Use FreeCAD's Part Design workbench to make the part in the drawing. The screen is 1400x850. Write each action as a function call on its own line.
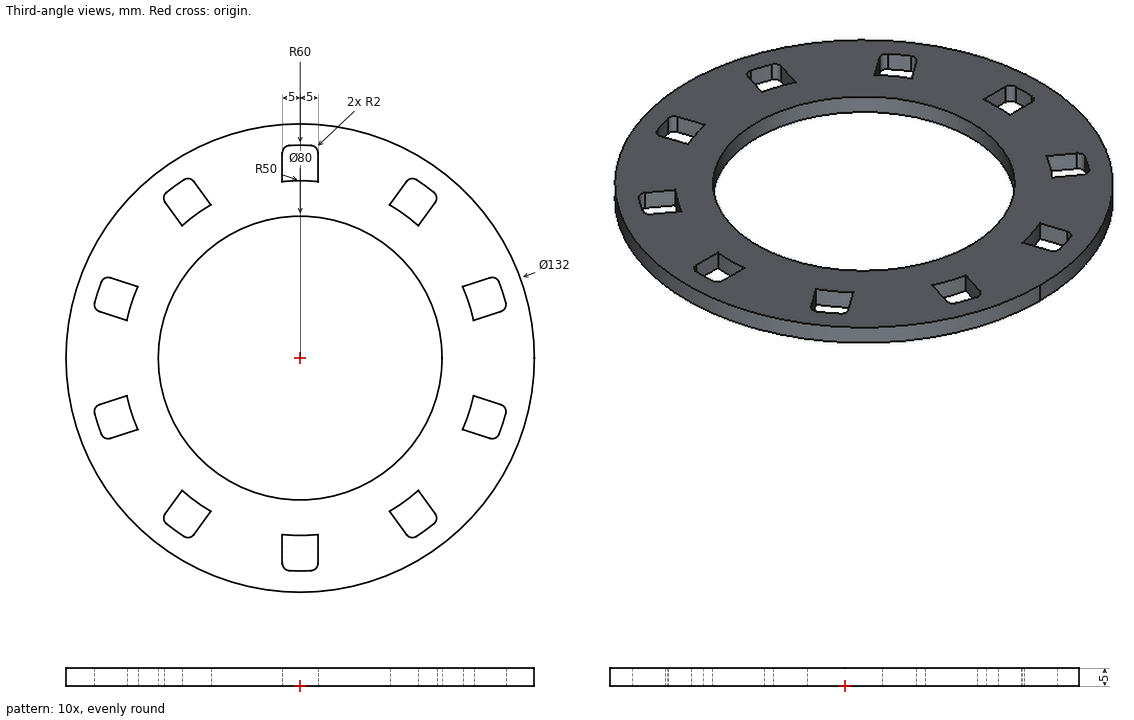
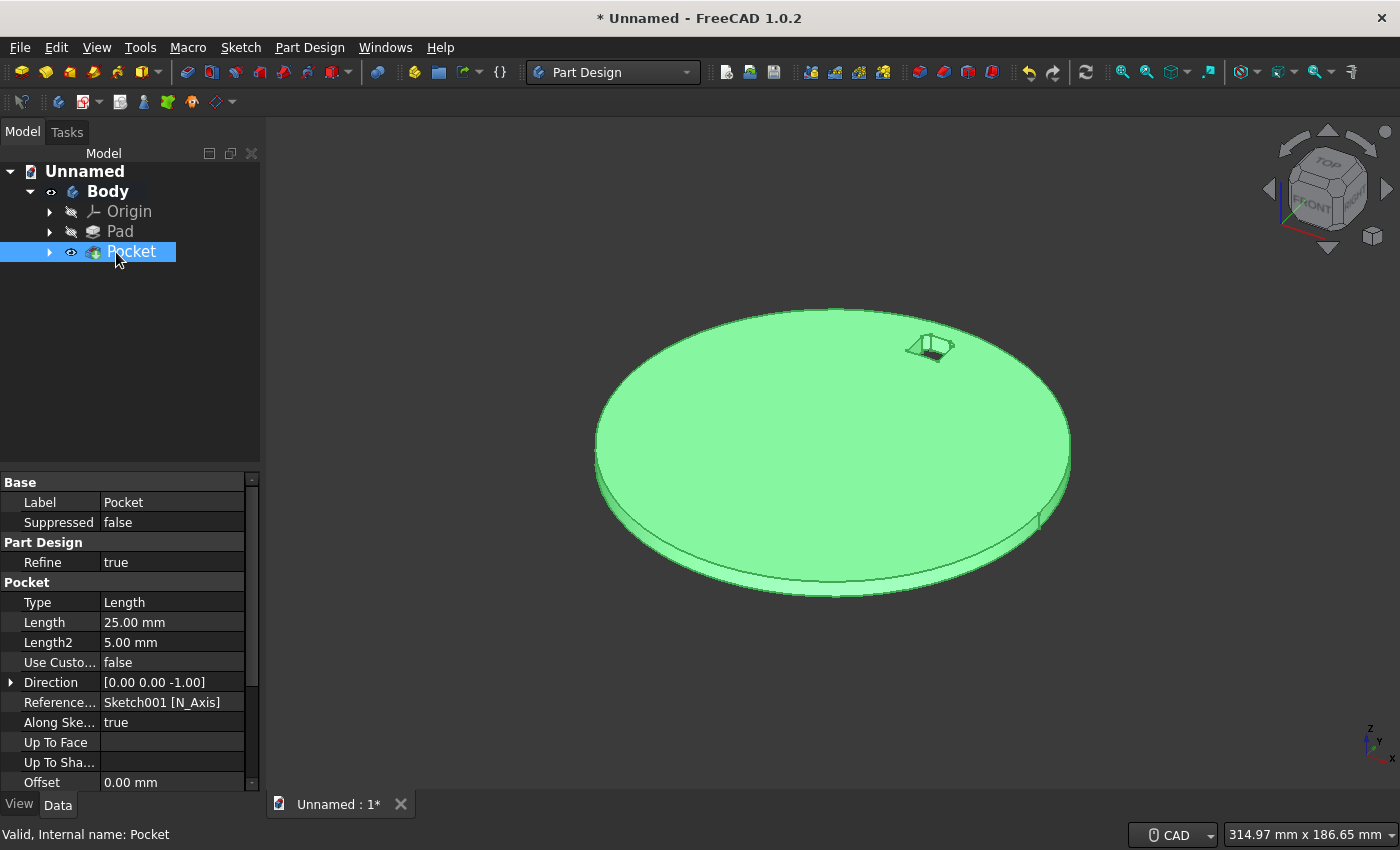
click(860, 72)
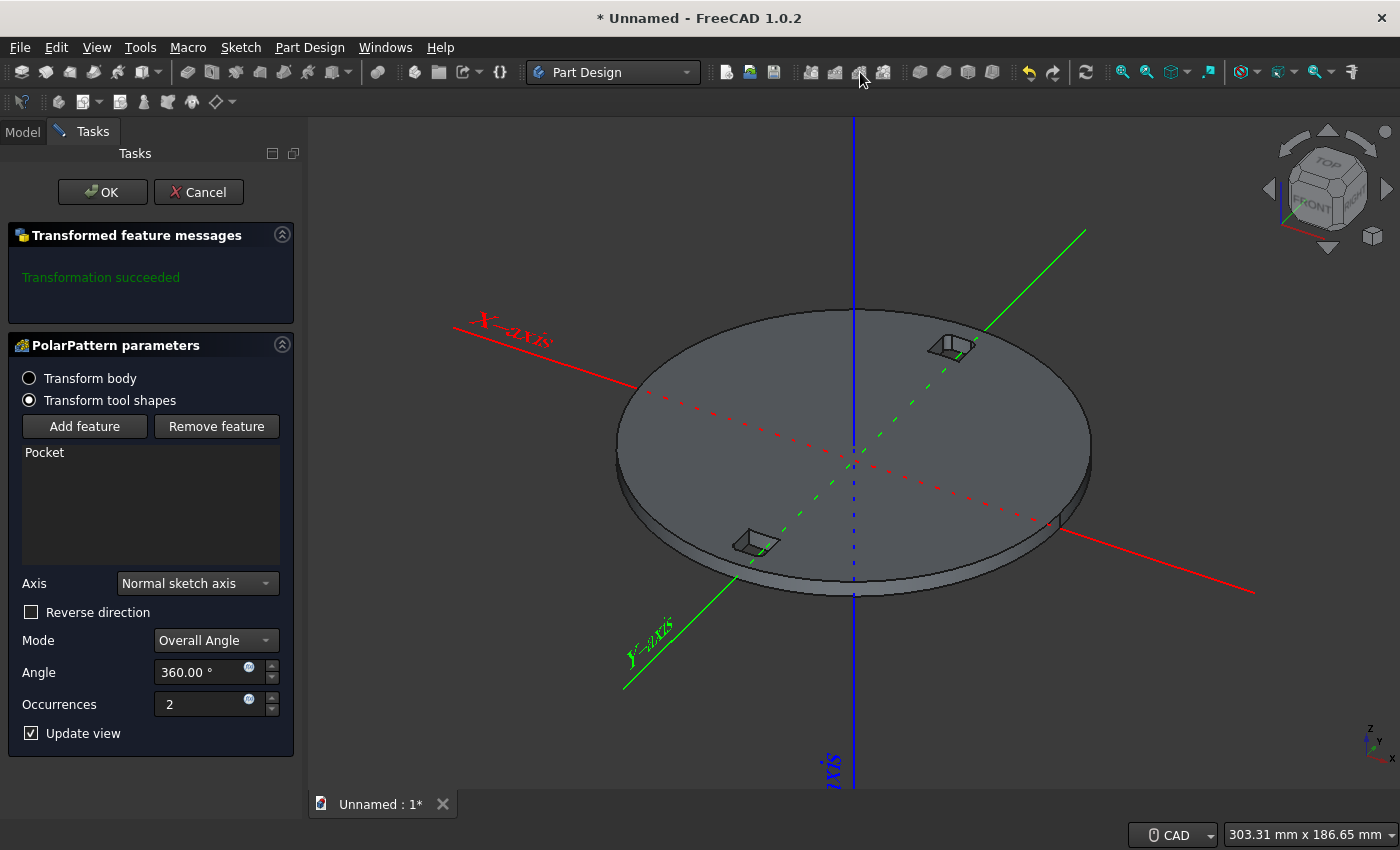
click(198, 584)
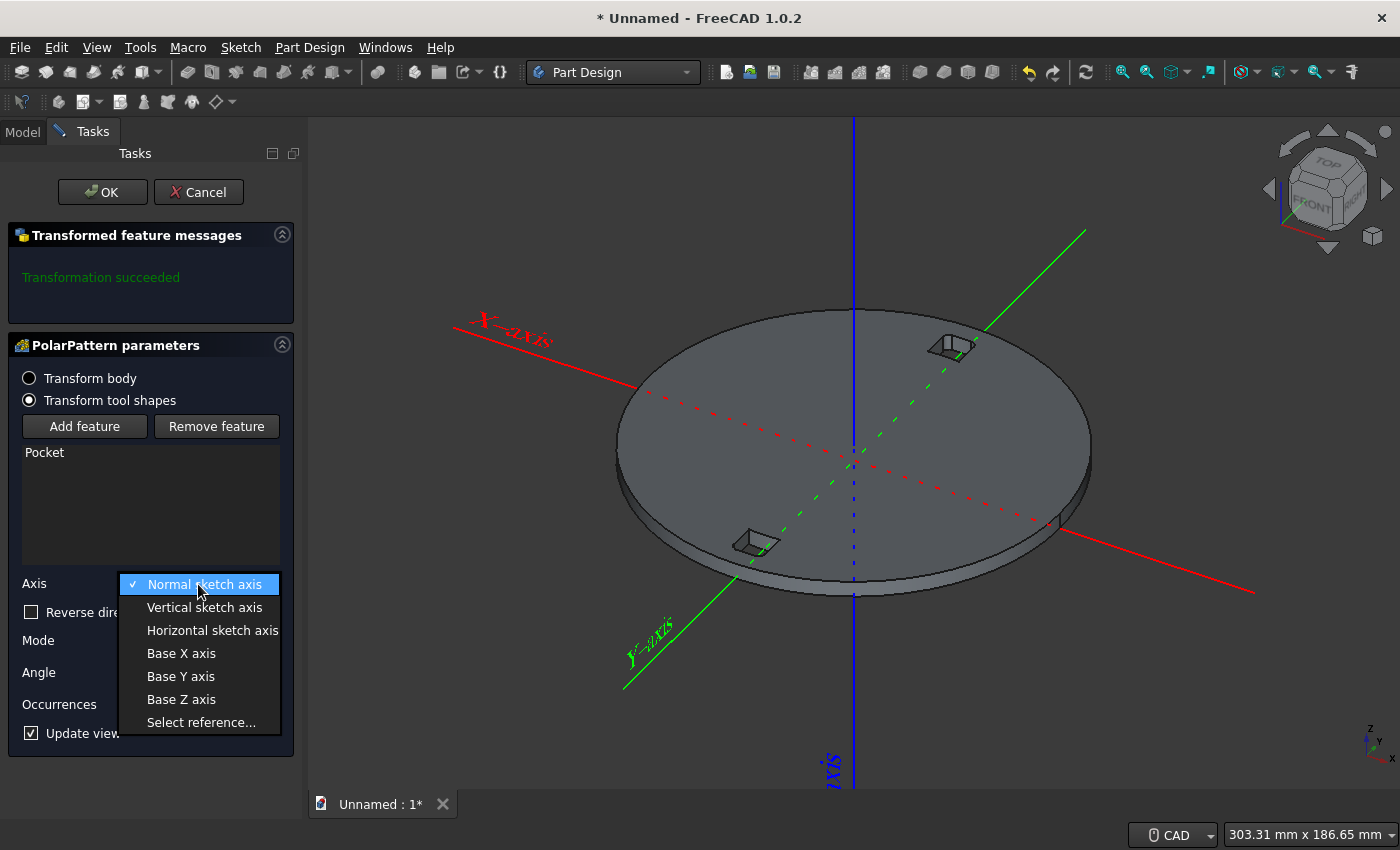
click(198, 700)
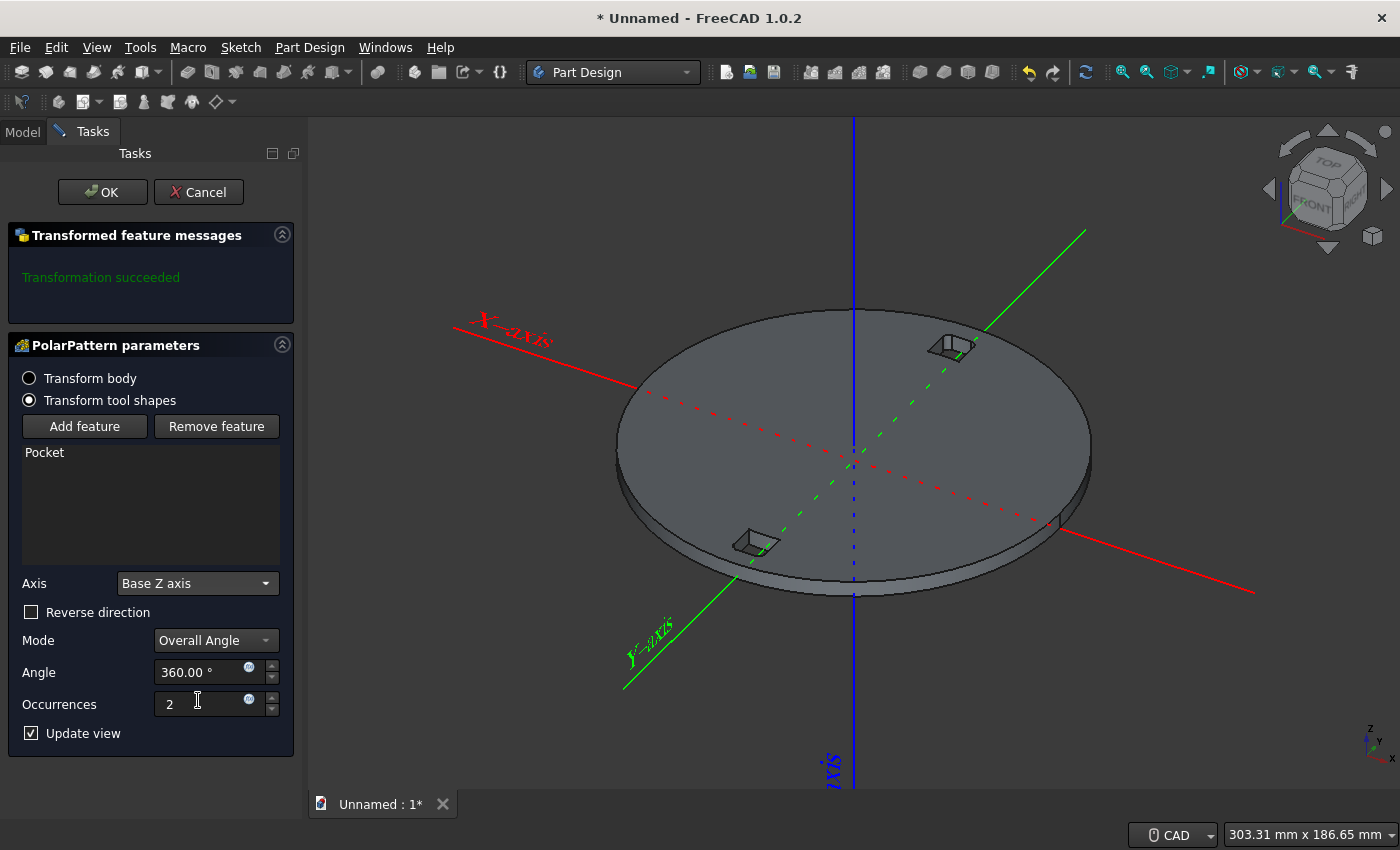
triple_click(209, 704)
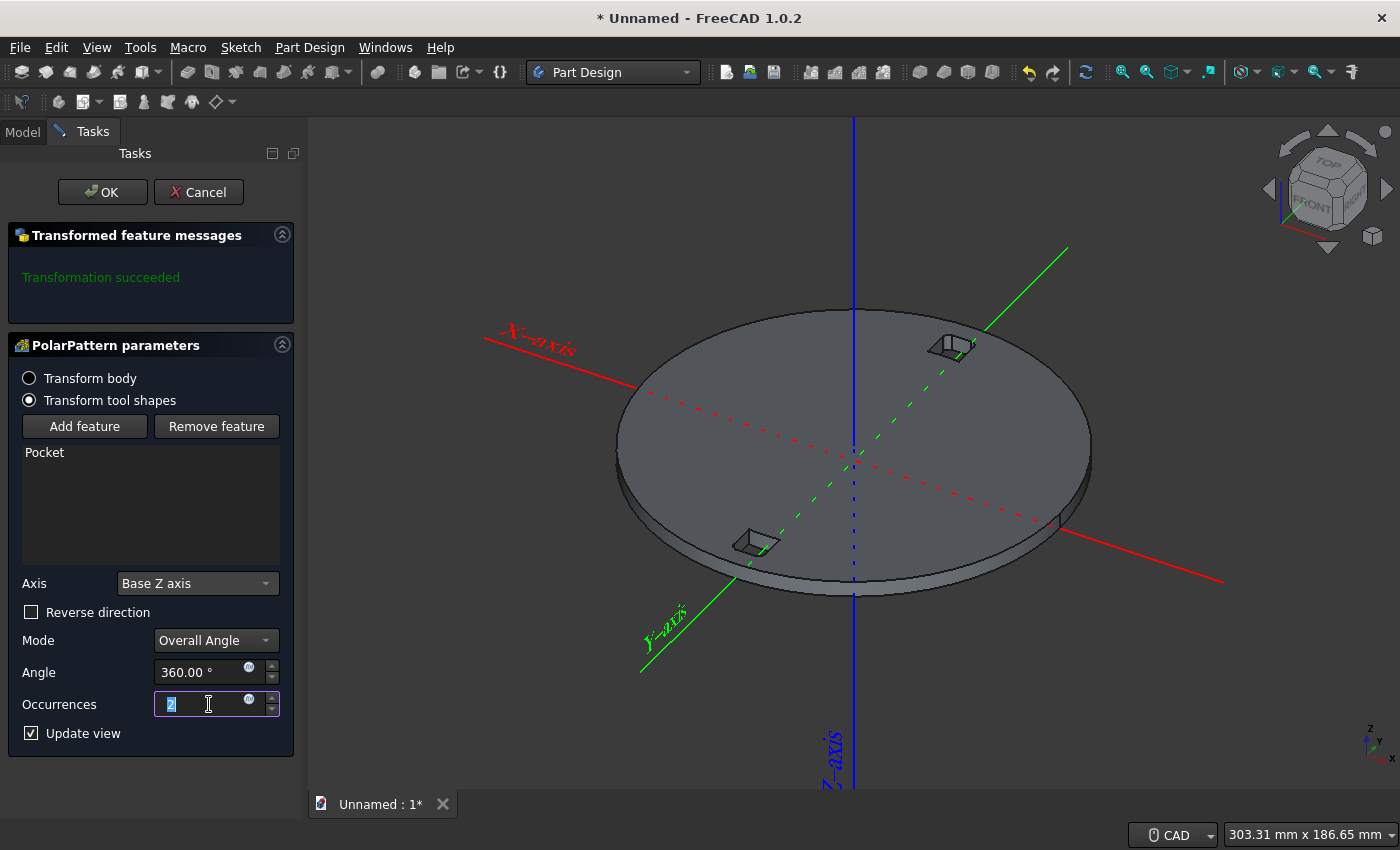
text(10)
key(Tab)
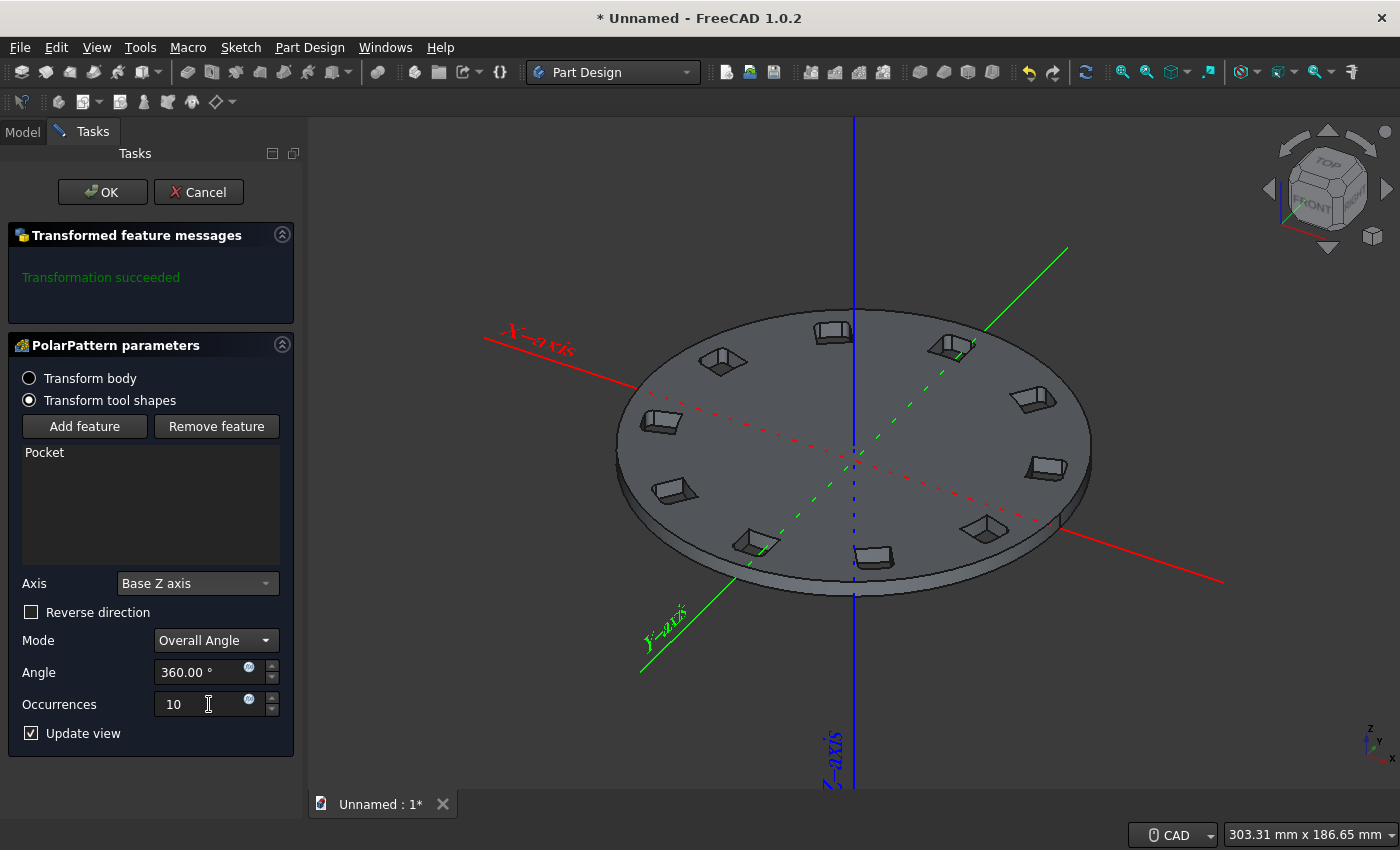
click(103, 192)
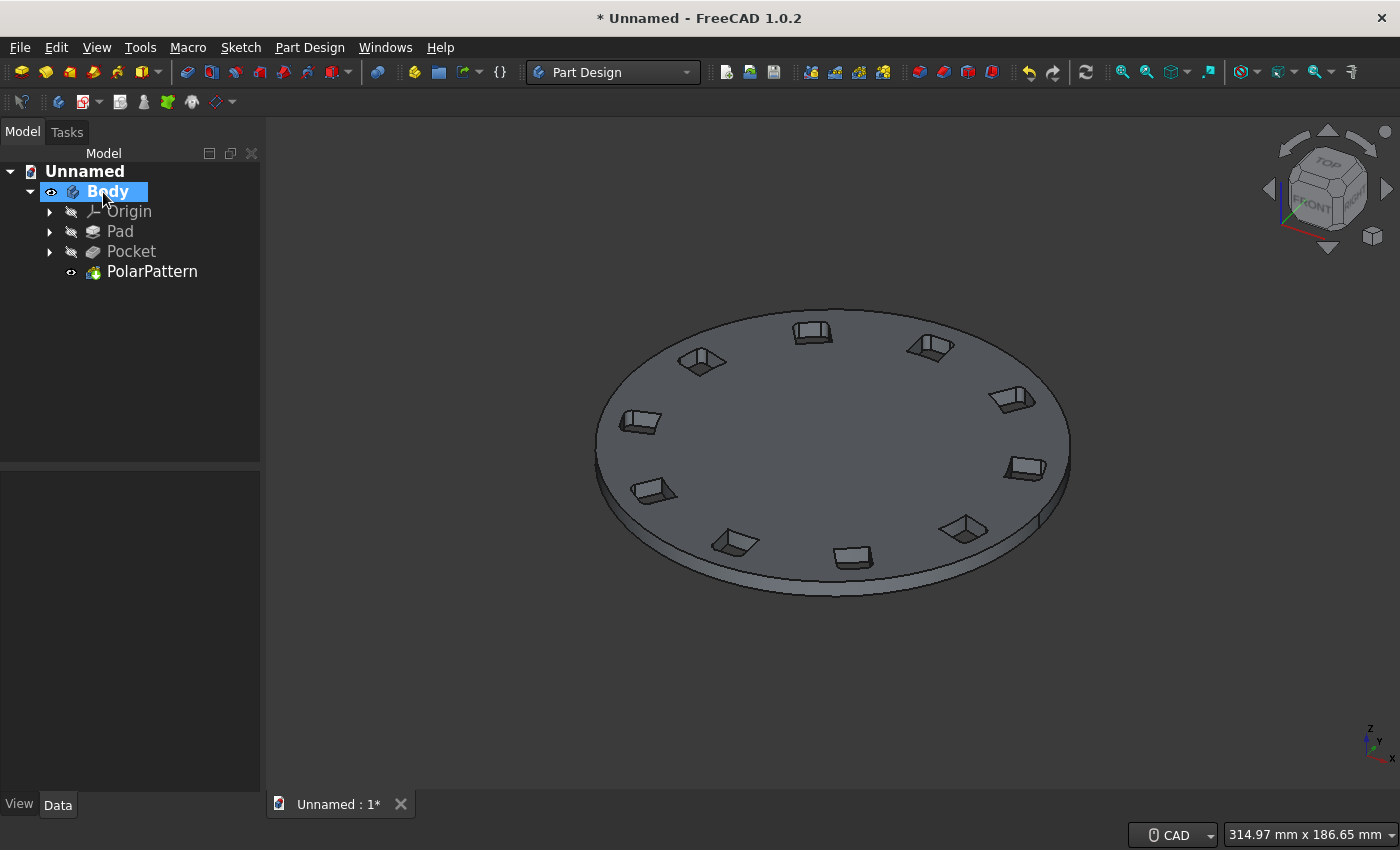
click(833, 445)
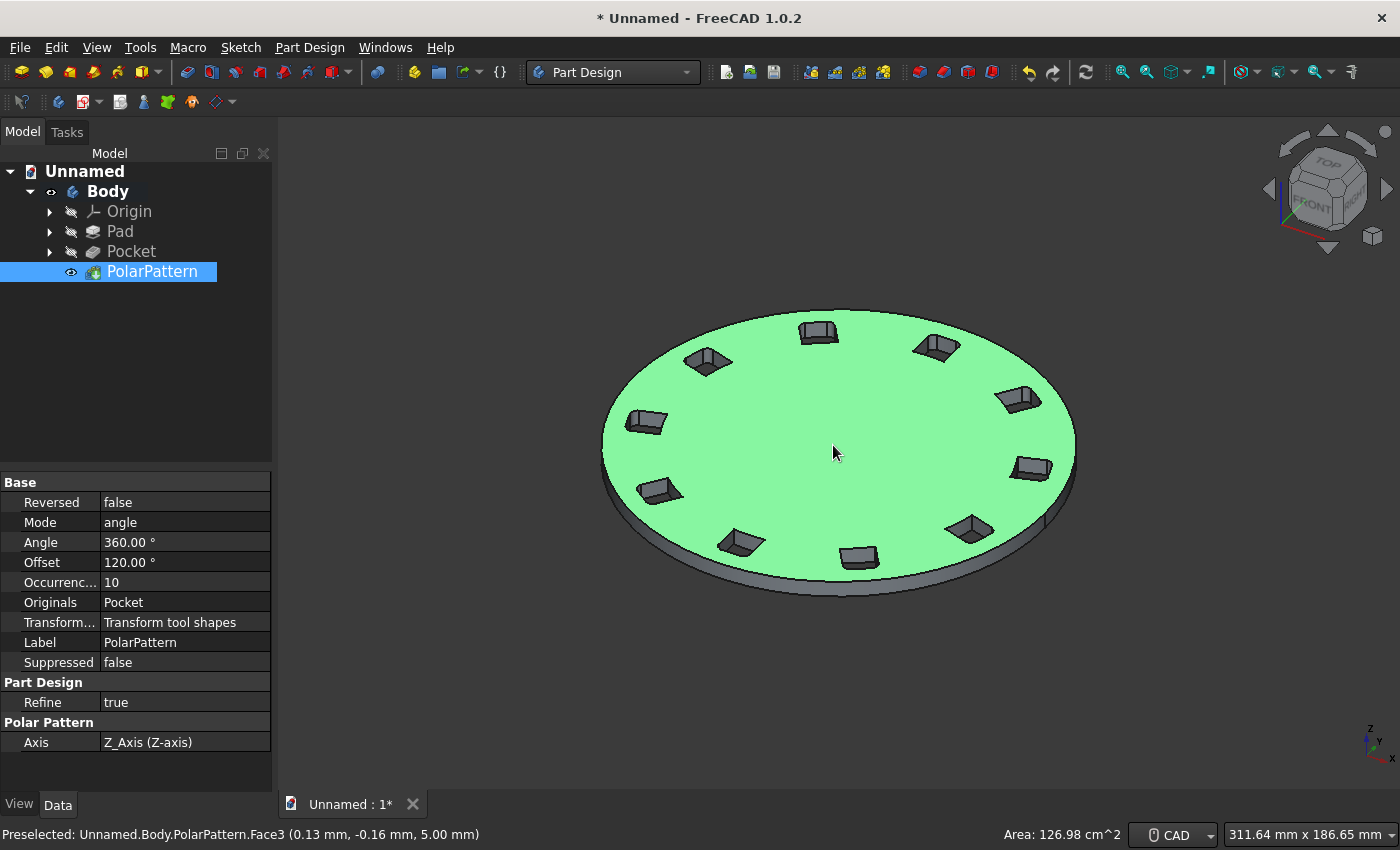
click(84, 102)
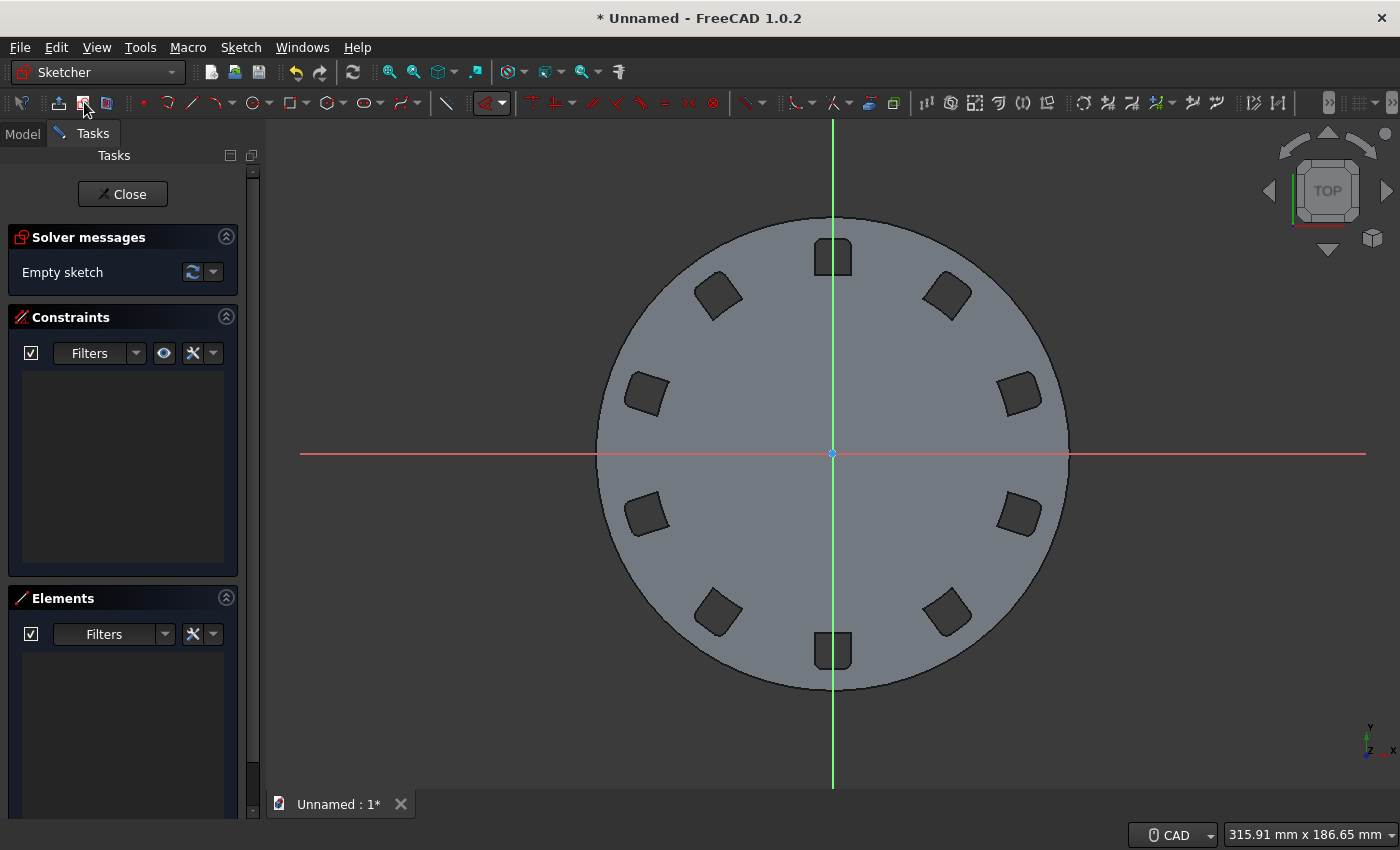
scroll(972, 454, up, 2)